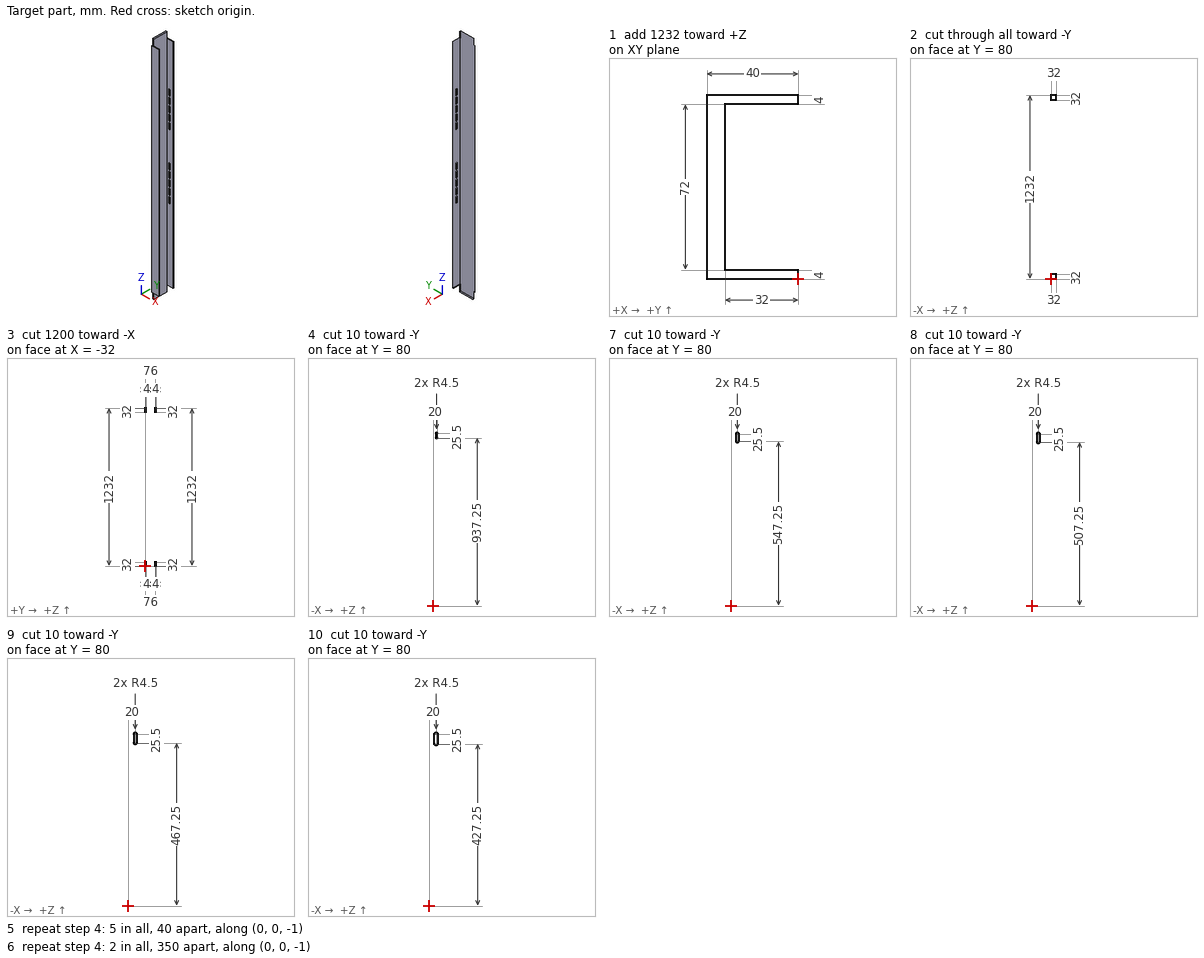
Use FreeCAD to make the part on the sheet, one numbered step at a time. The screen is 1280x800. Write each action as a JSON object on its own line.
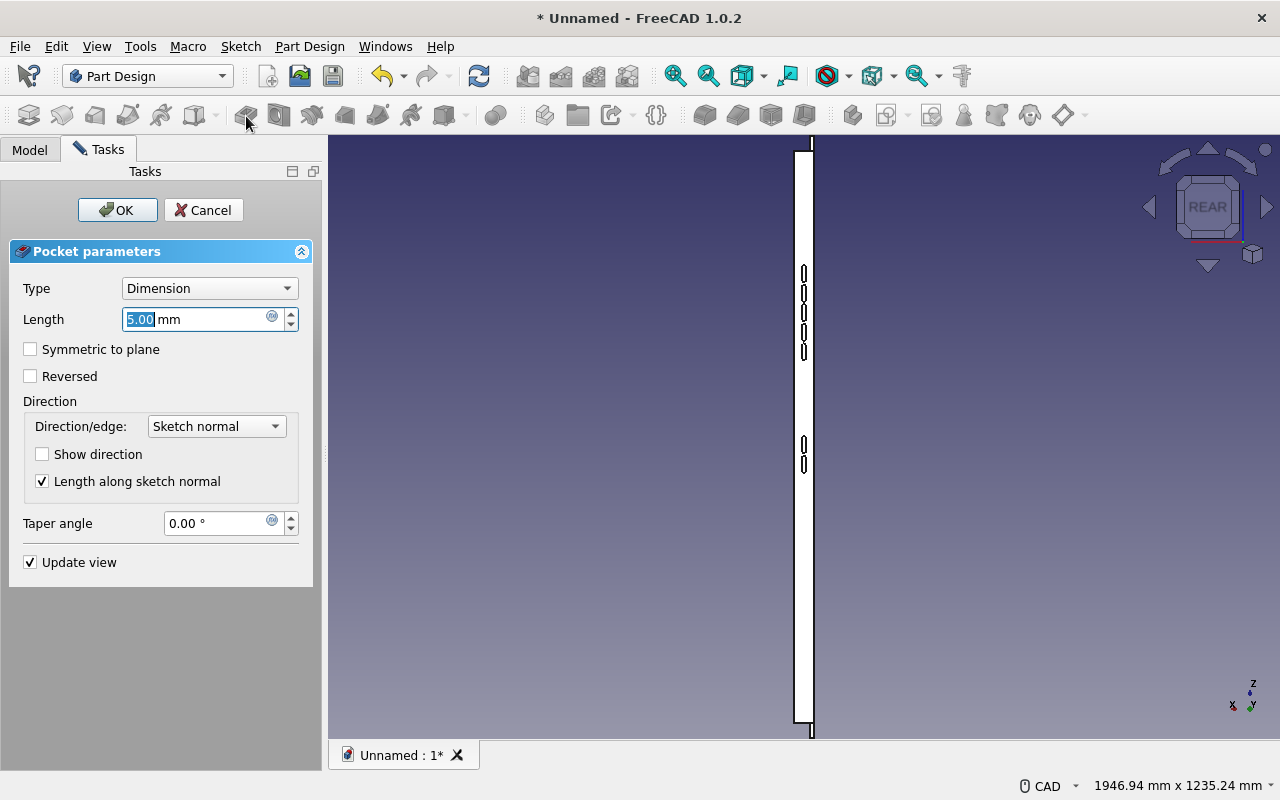
{"action": "type", "text": "10"}
{"action": "key", "text": "Tab"}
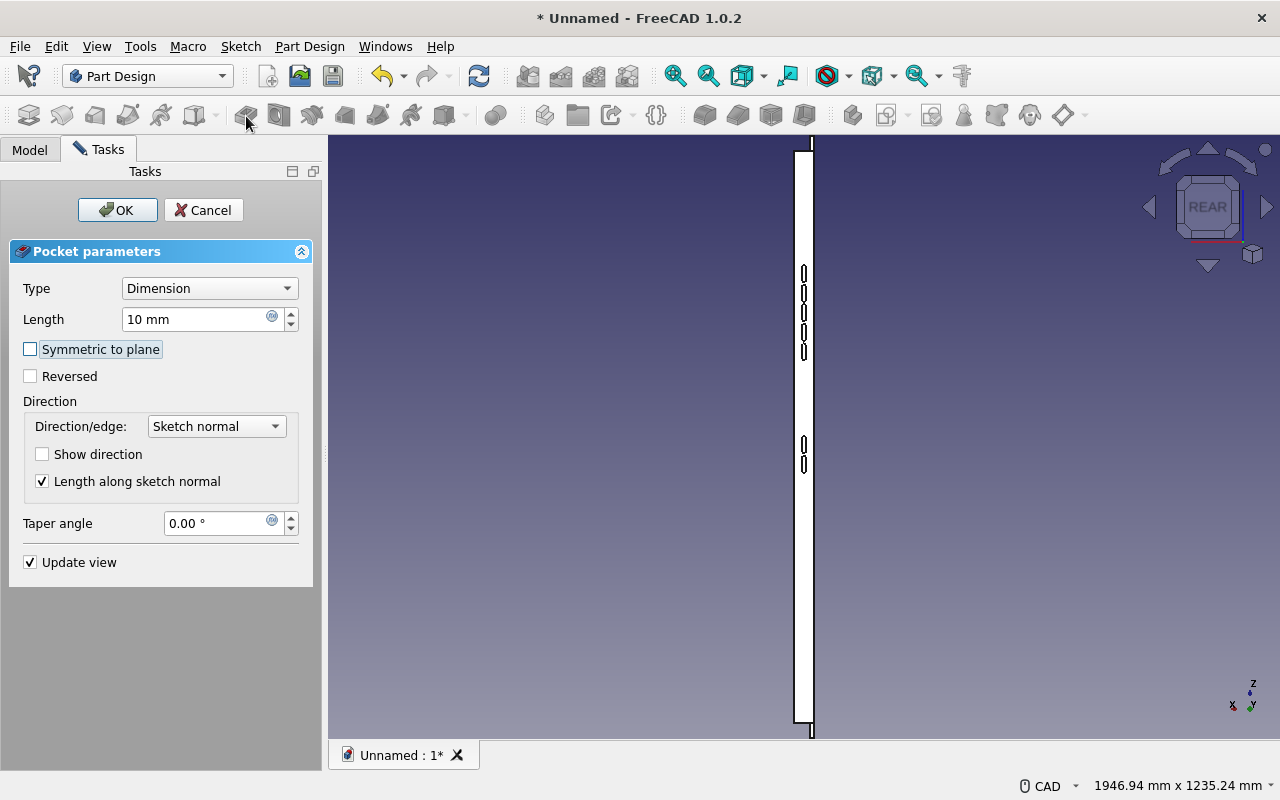
{"action": "left_click", "coordinate": [118, 210]}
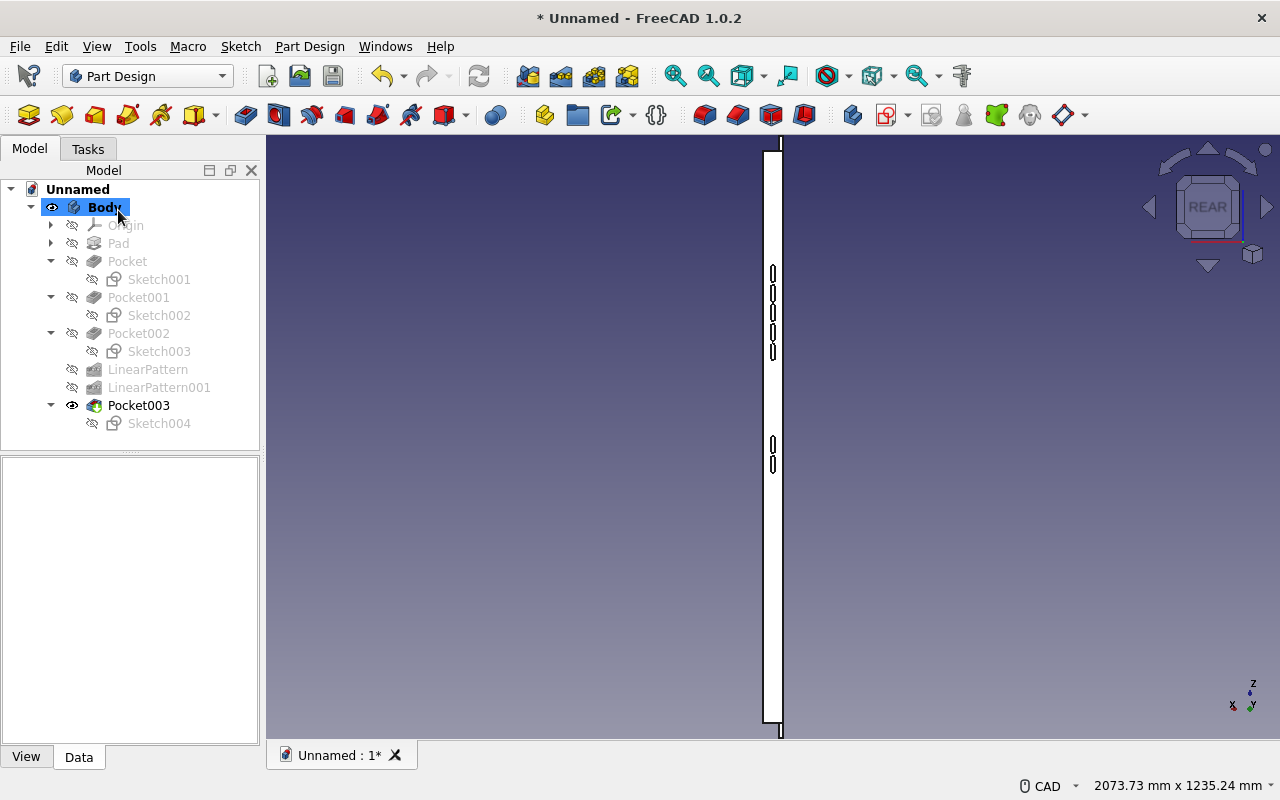
{"action": "left_click", "coordinate": [773, 191]}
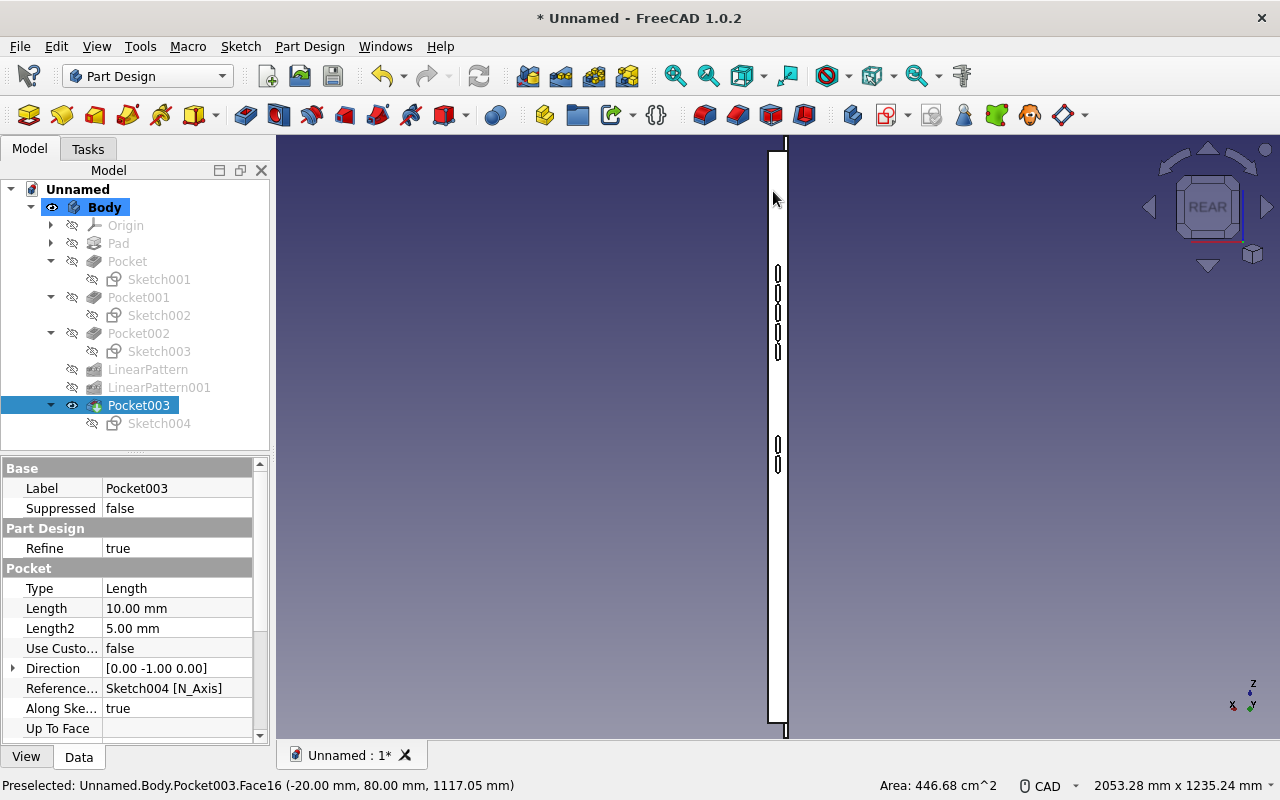
{"action": "left_click", "coordinate": [886, 116]}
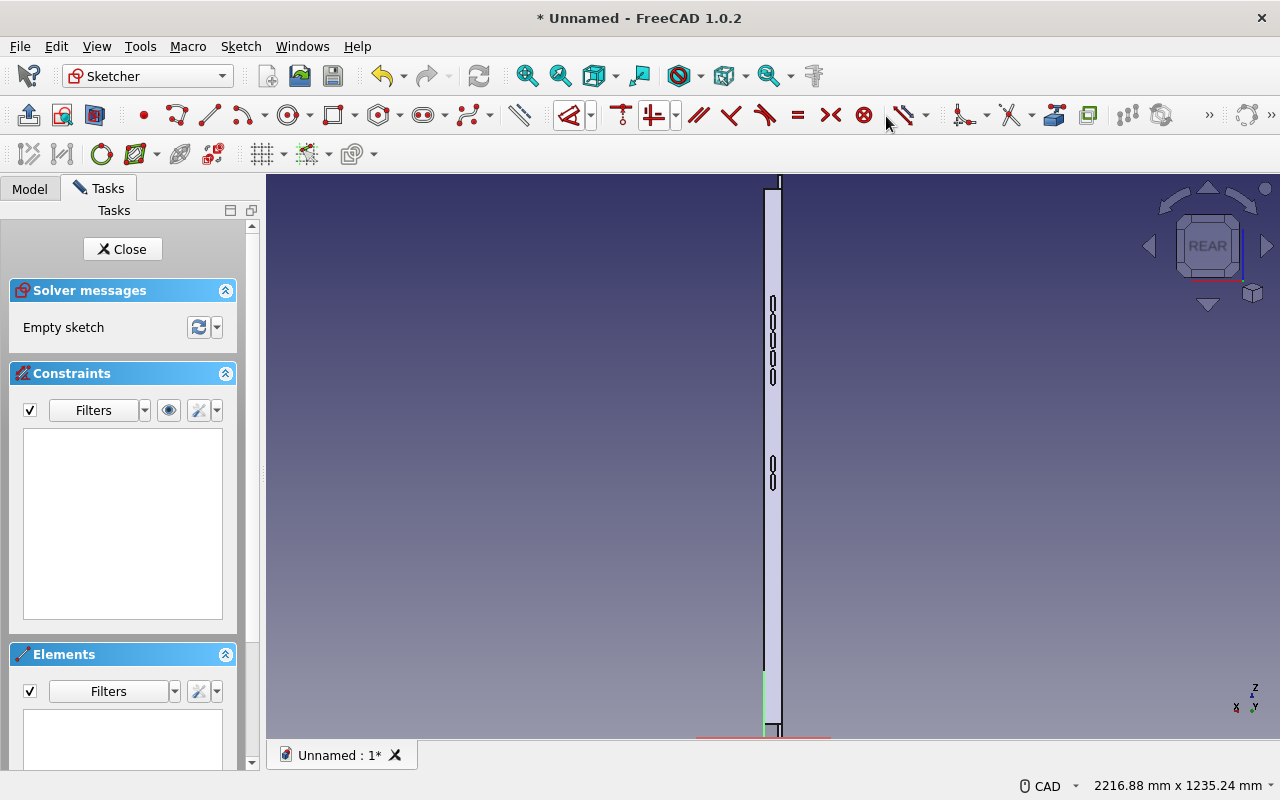
{"action": "scroll", "coordinate": [777, 503], "scroll_direction": "up", "scroll_amount": 15}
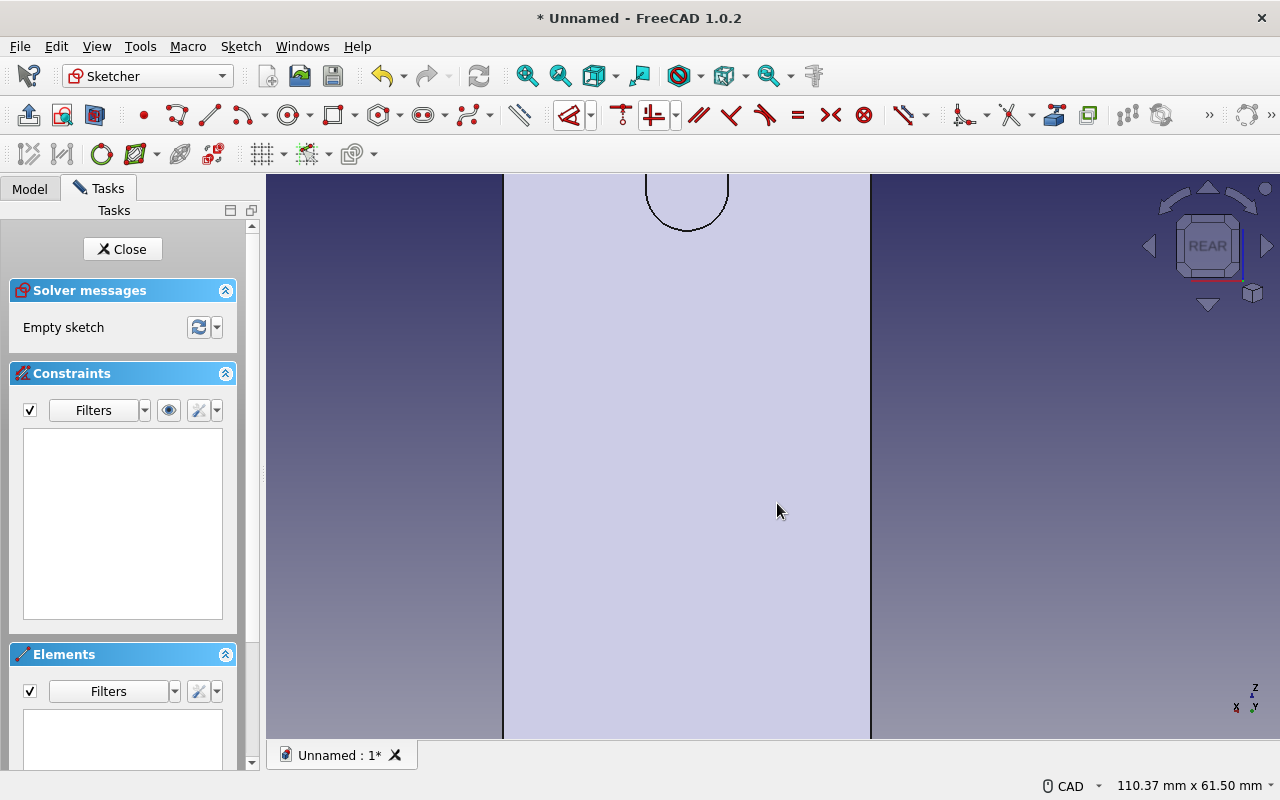
{"action": "left_click", "coordinate": [422, 116]}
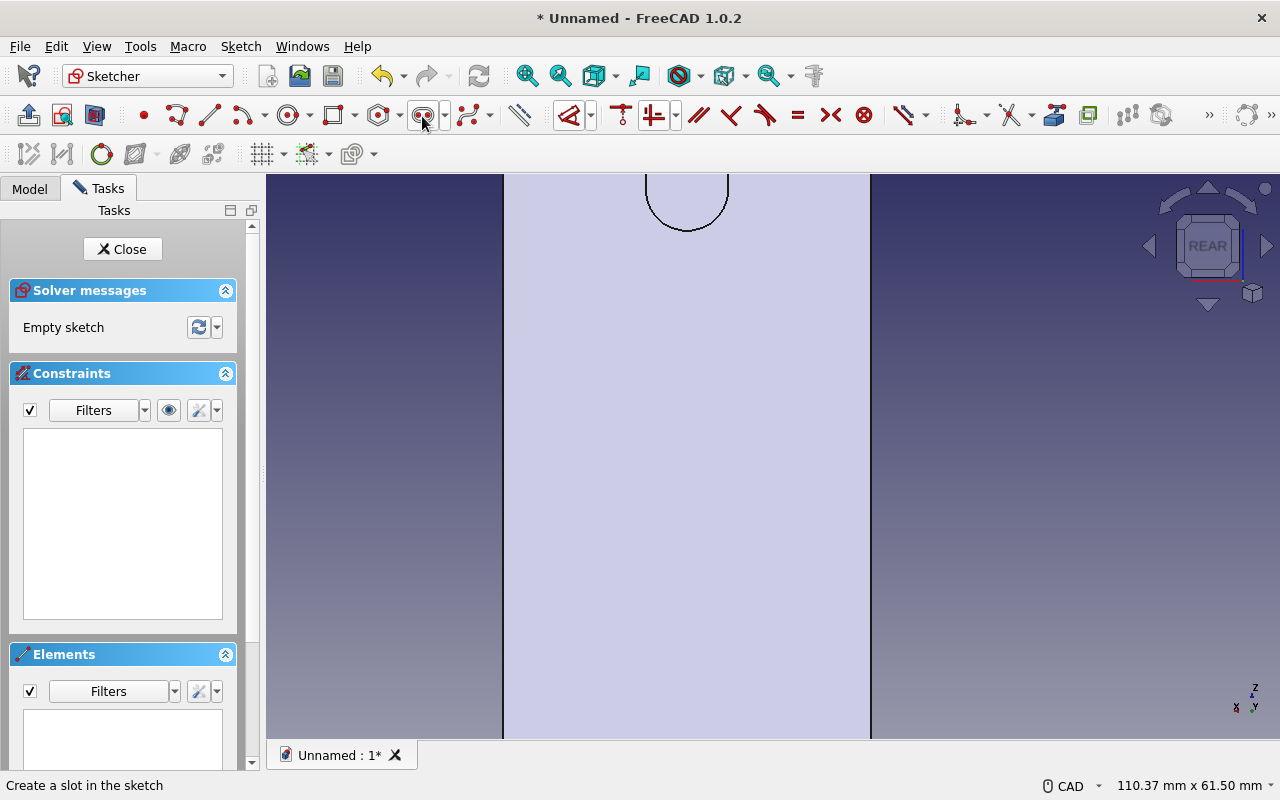
{"action": "left_click", "coordinate": [687, 557]}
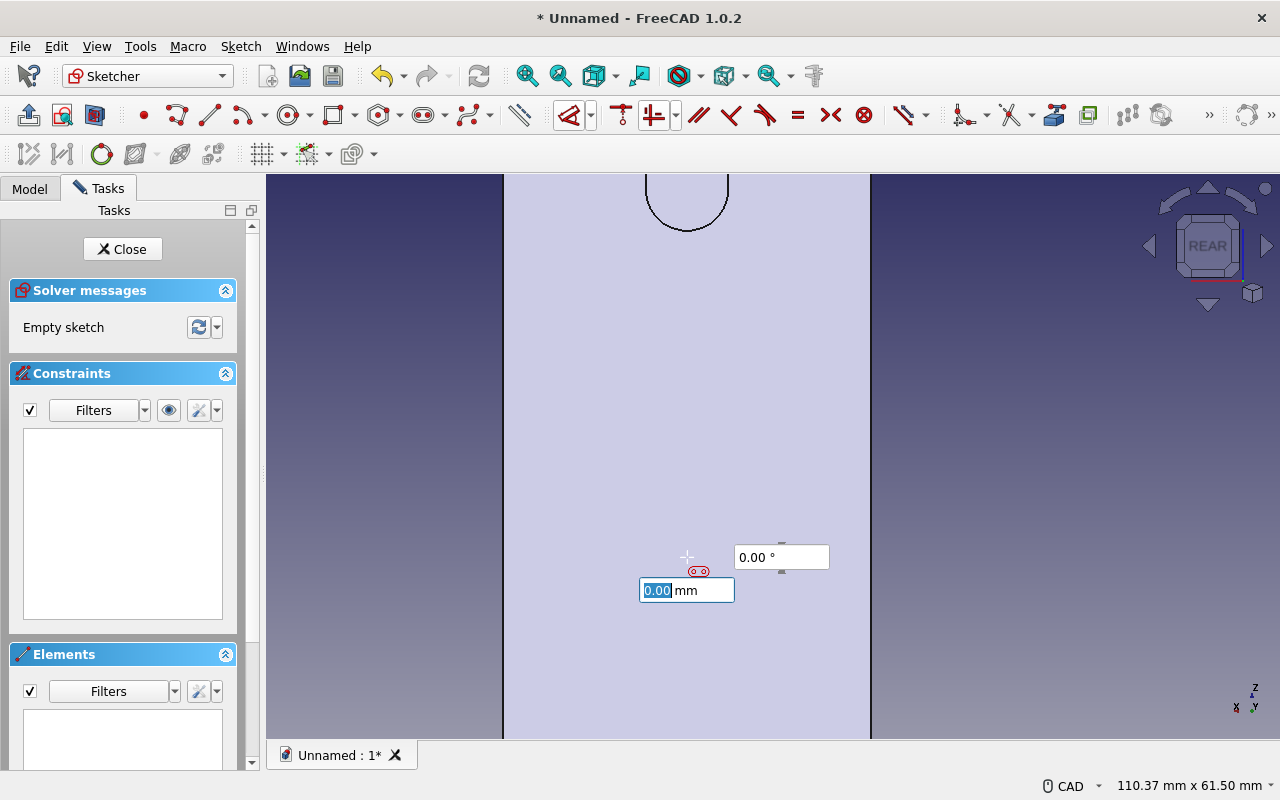
{"action": "left_click", "coordinate": [687, 323]}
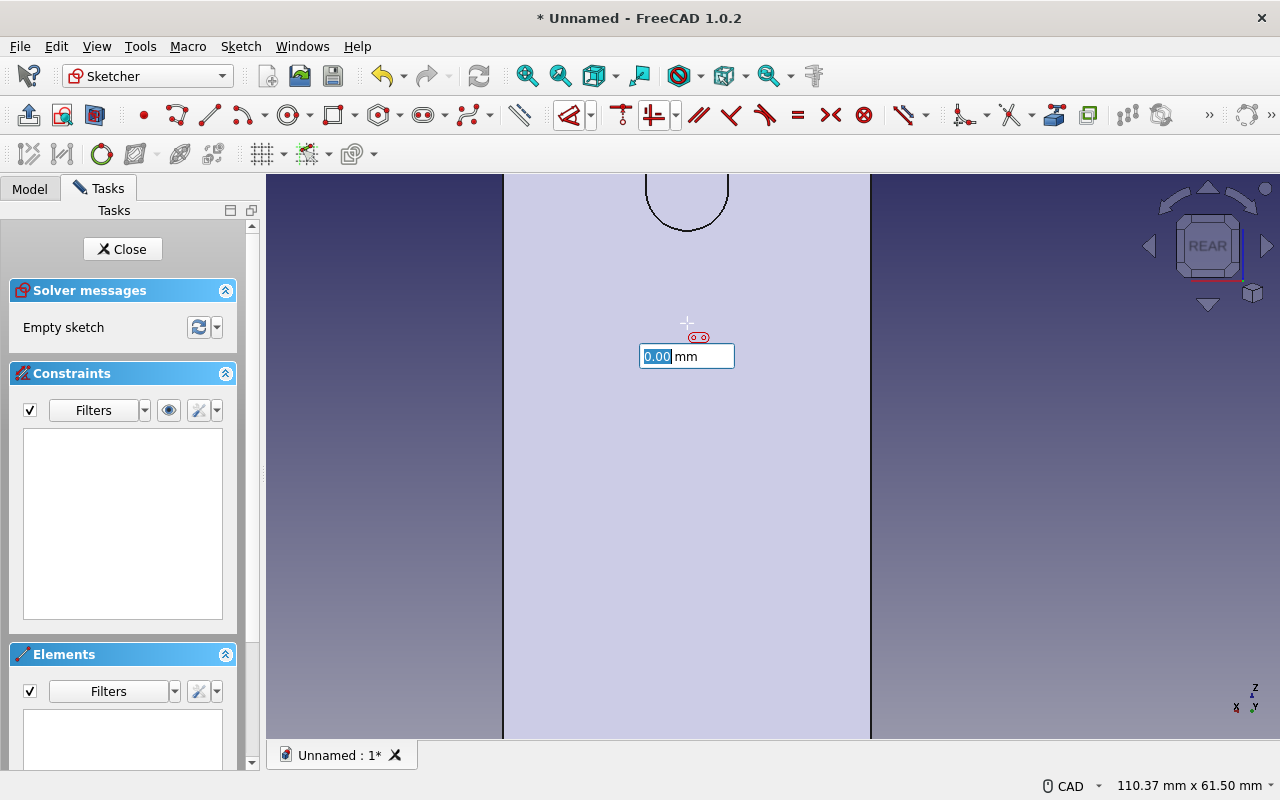
{"action": "left_click", "coordinate": [728, 440]}
{"action": "key", "text": "Escape"}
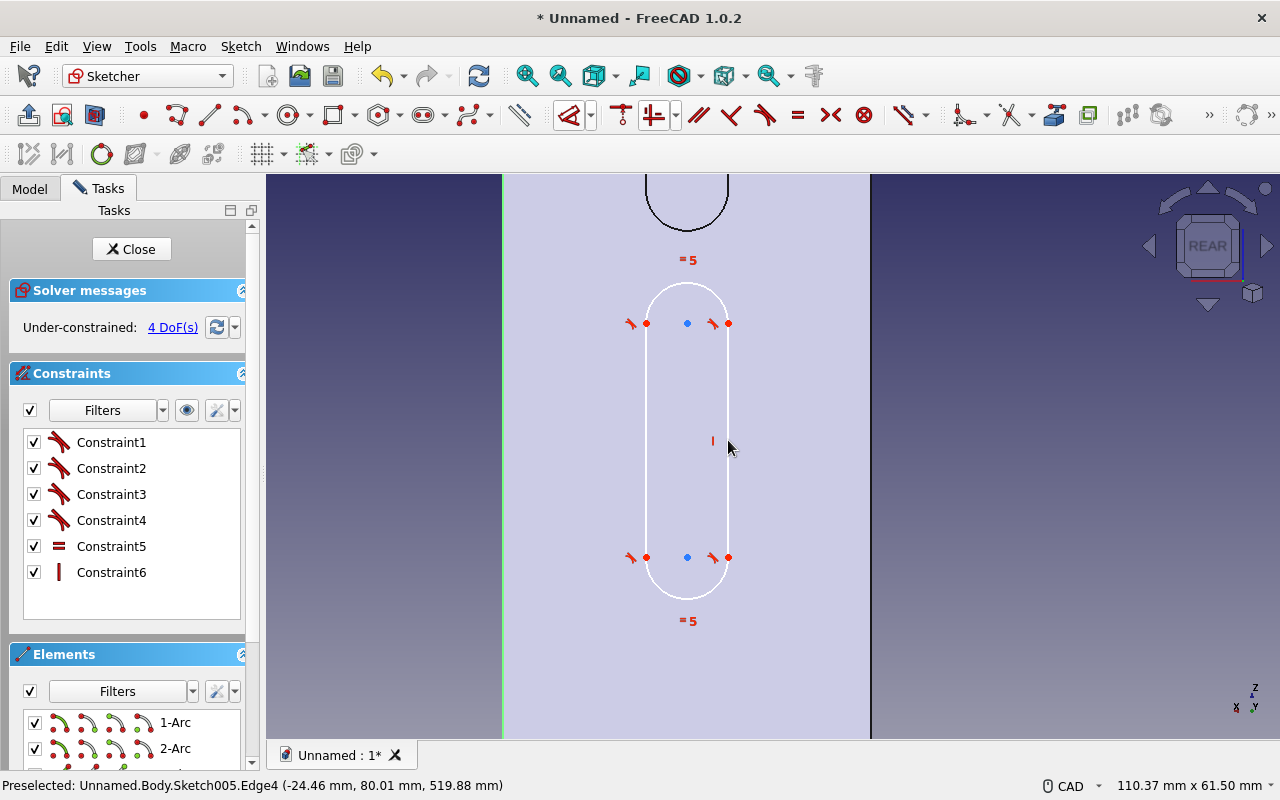
{"action": "left_click", "coordinate": [663, 591]}